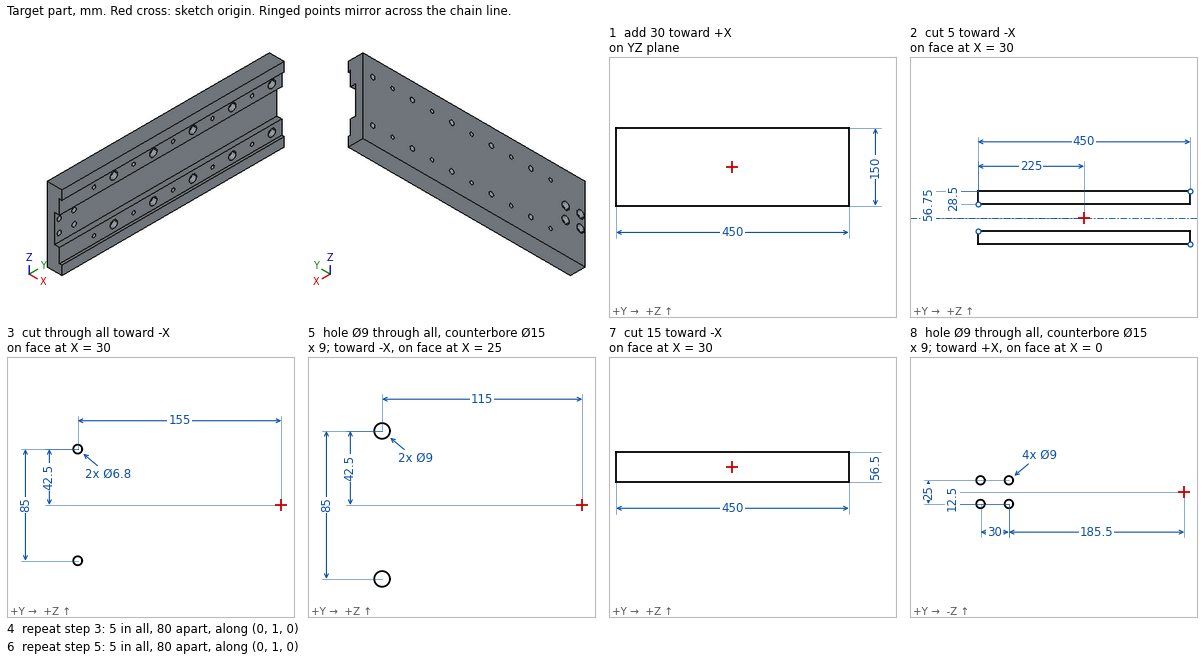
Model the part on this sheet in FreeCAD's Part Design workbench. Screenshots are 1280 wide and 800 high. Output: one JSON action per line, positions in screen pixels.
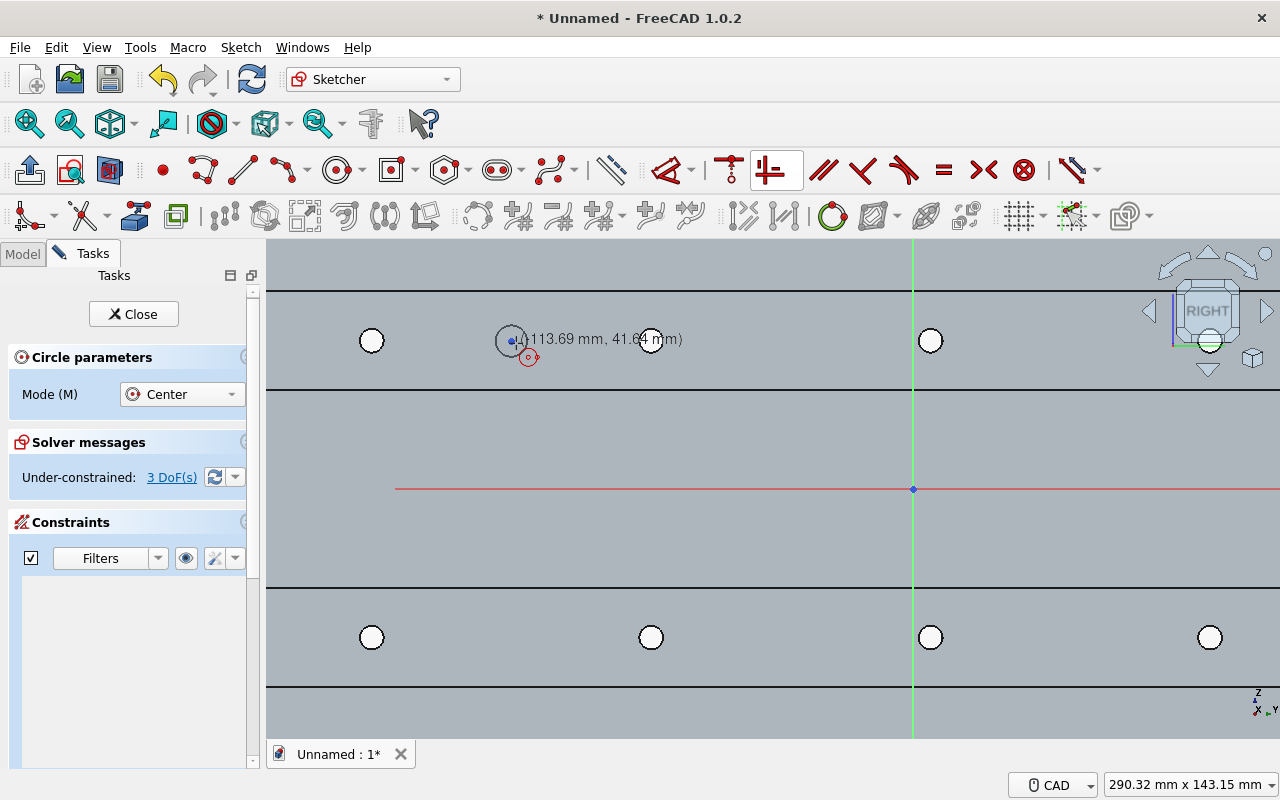
{"action": "scroll", "coordinate": [511, 638], "scroll_direction": "up", "scroll_amount": 2}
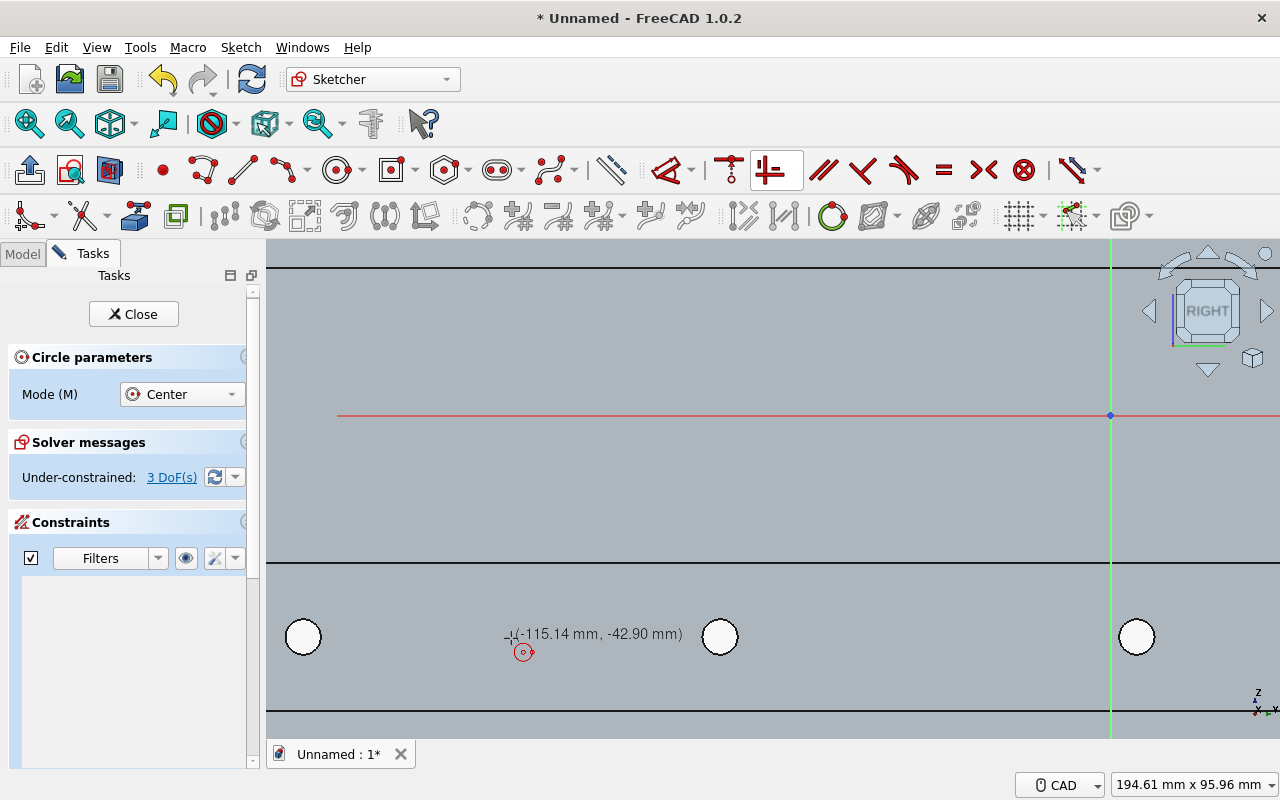
{"action": "left_click", "coordinate": [512, 637]}
{"action": "left_click", "coordinate": [528, 620]}
{"action": "key", "text": "Escape"}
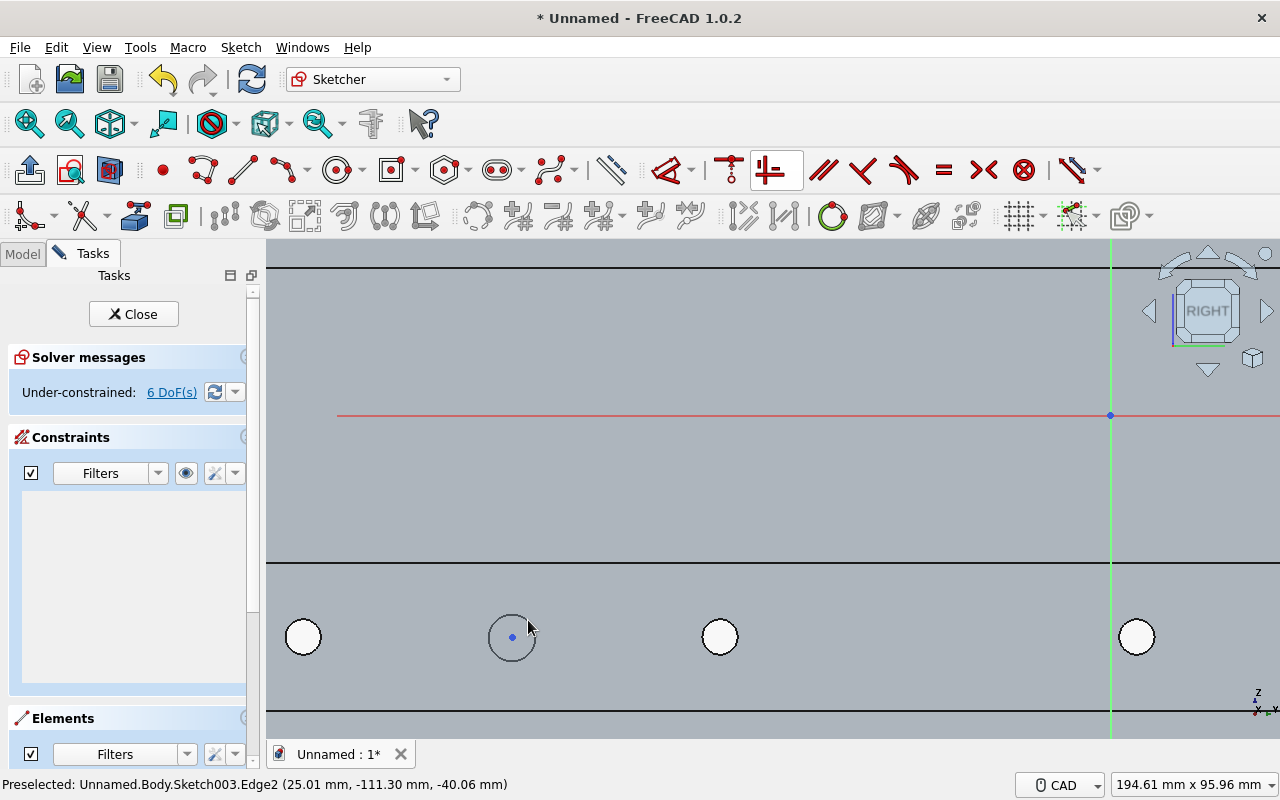
{"action": "scroll", "coordinate": [511, 638], "scroll_direction": "down", "scroll_amount": 2}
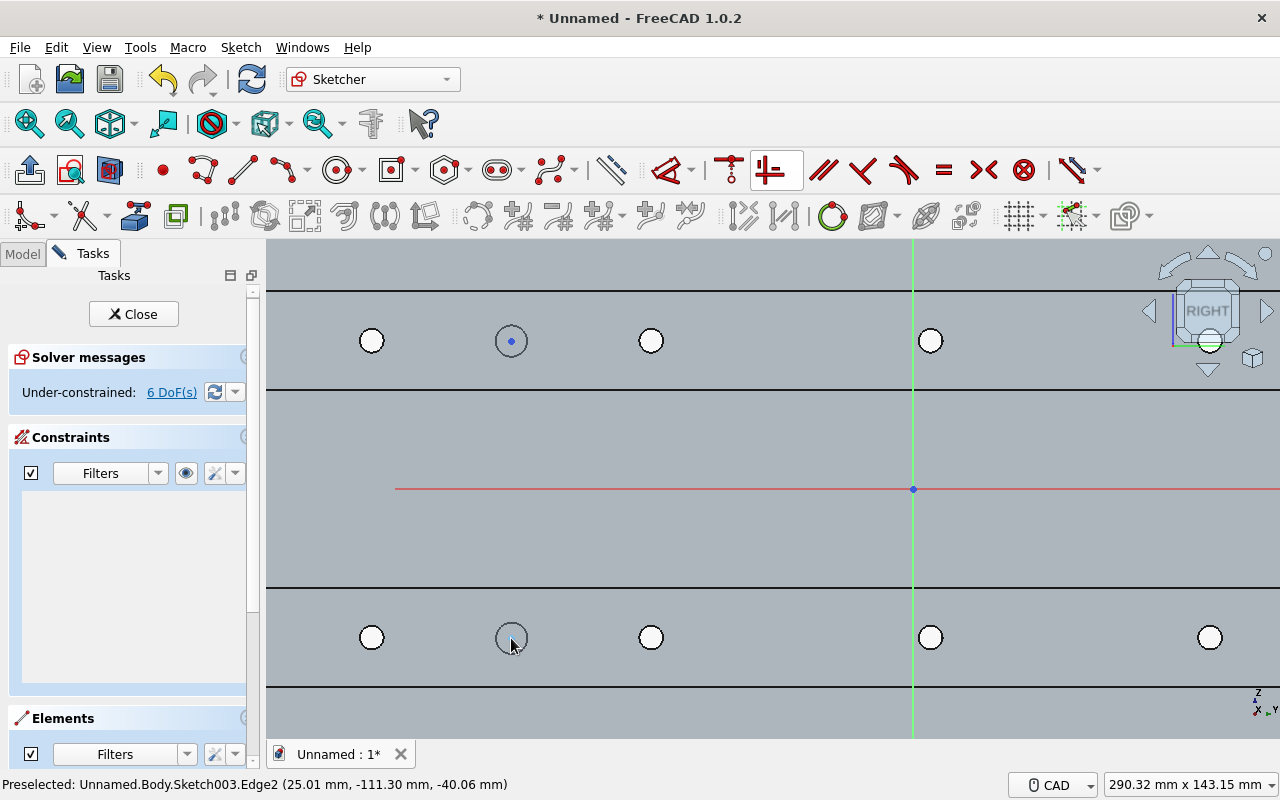
{"action": "left_click", "coordinate": [522, 330]}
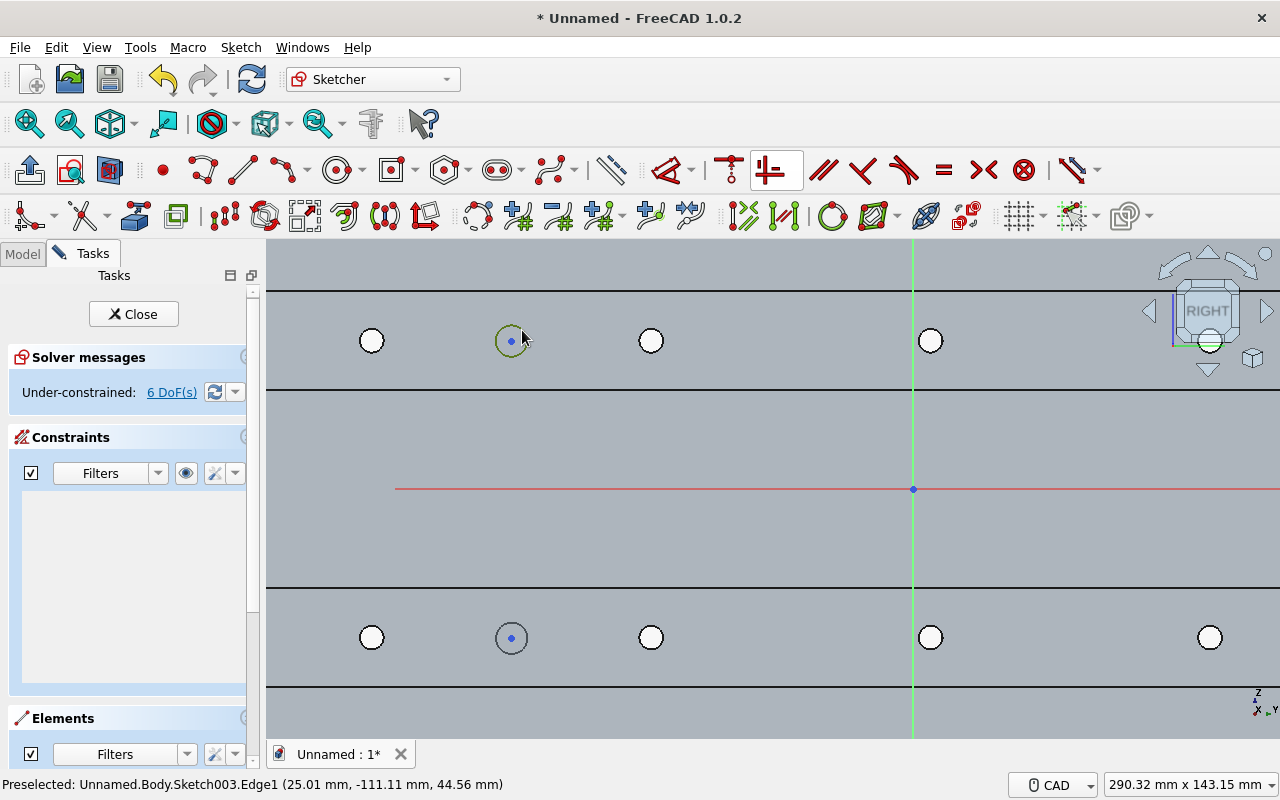
{"action": "left_click", "coordinate": [523, 627]}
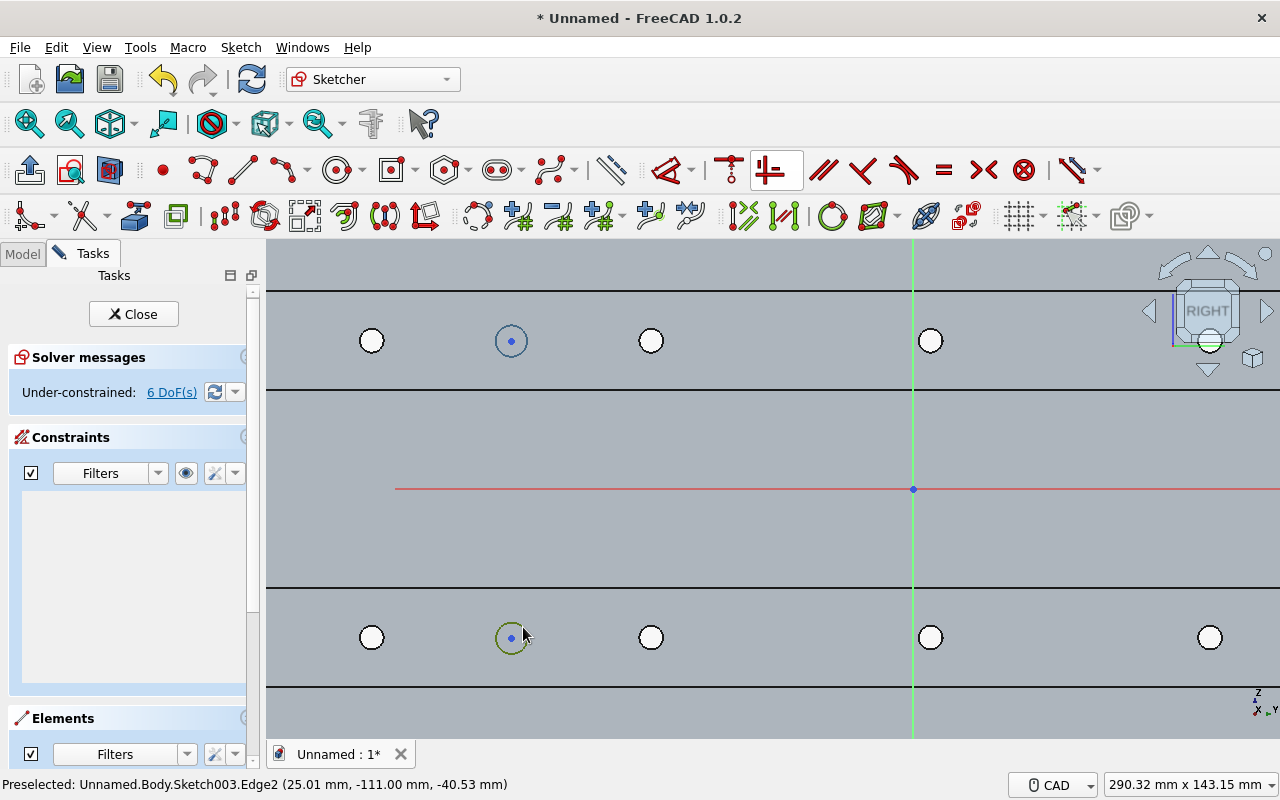
{"action": "left_click", "coordinate": [944, 170]}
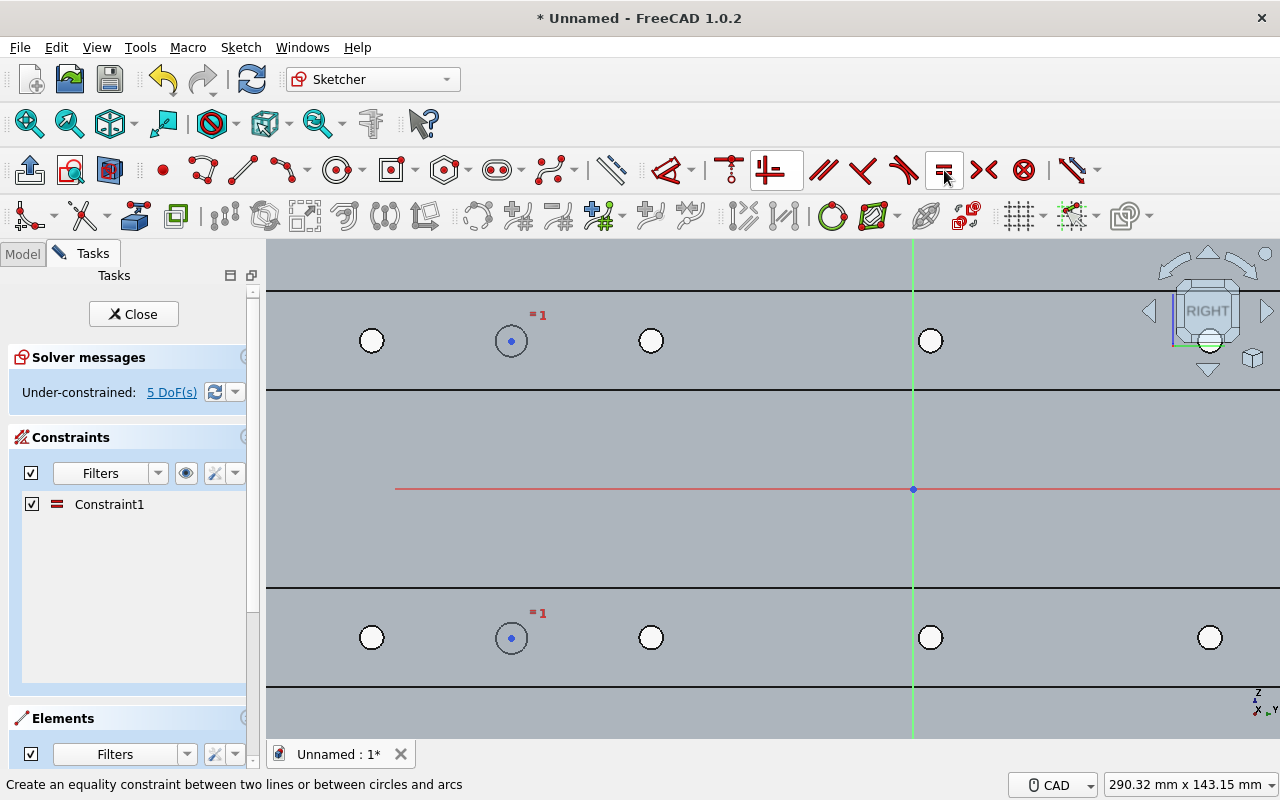
{"action": "left_click", "coordinate": [511, 341]}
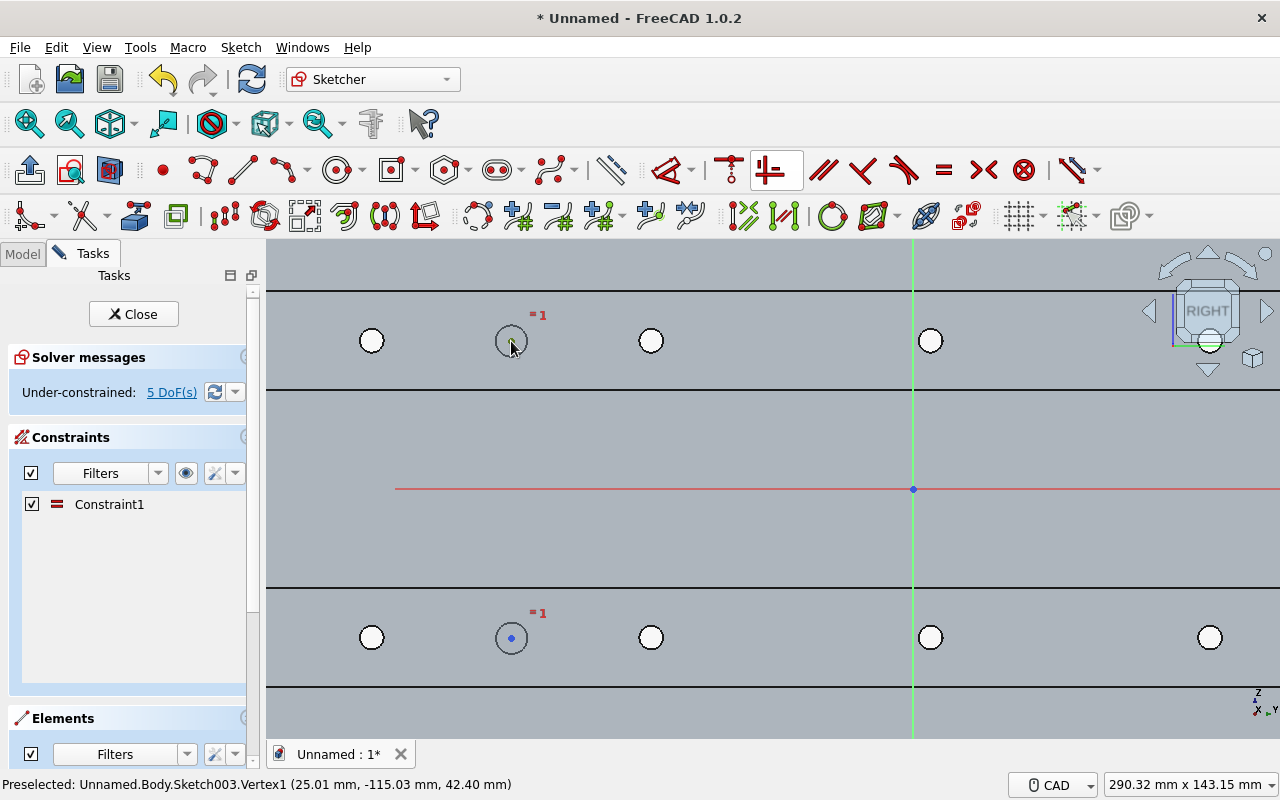
{"action": "left_click", "coordinate": [512, 638]}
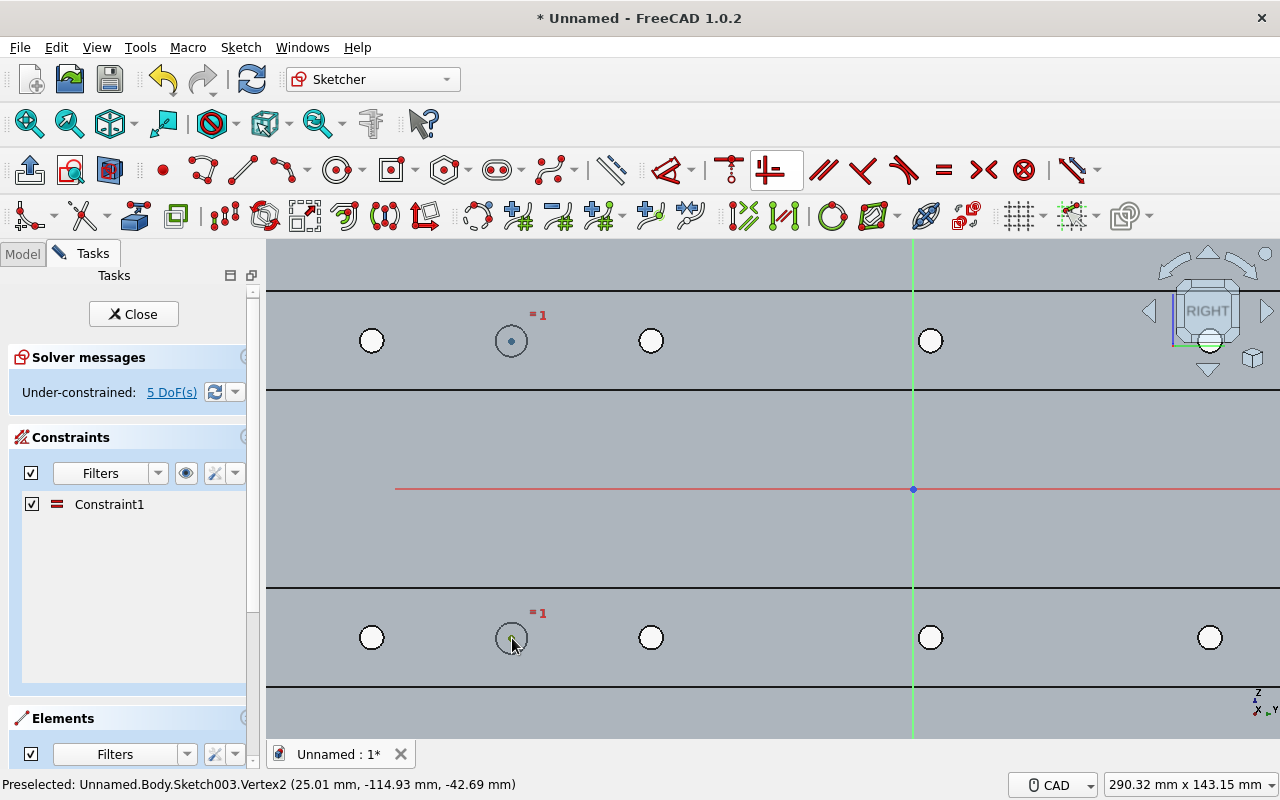
{"action": "left_click", "coordinate": [798, 170]}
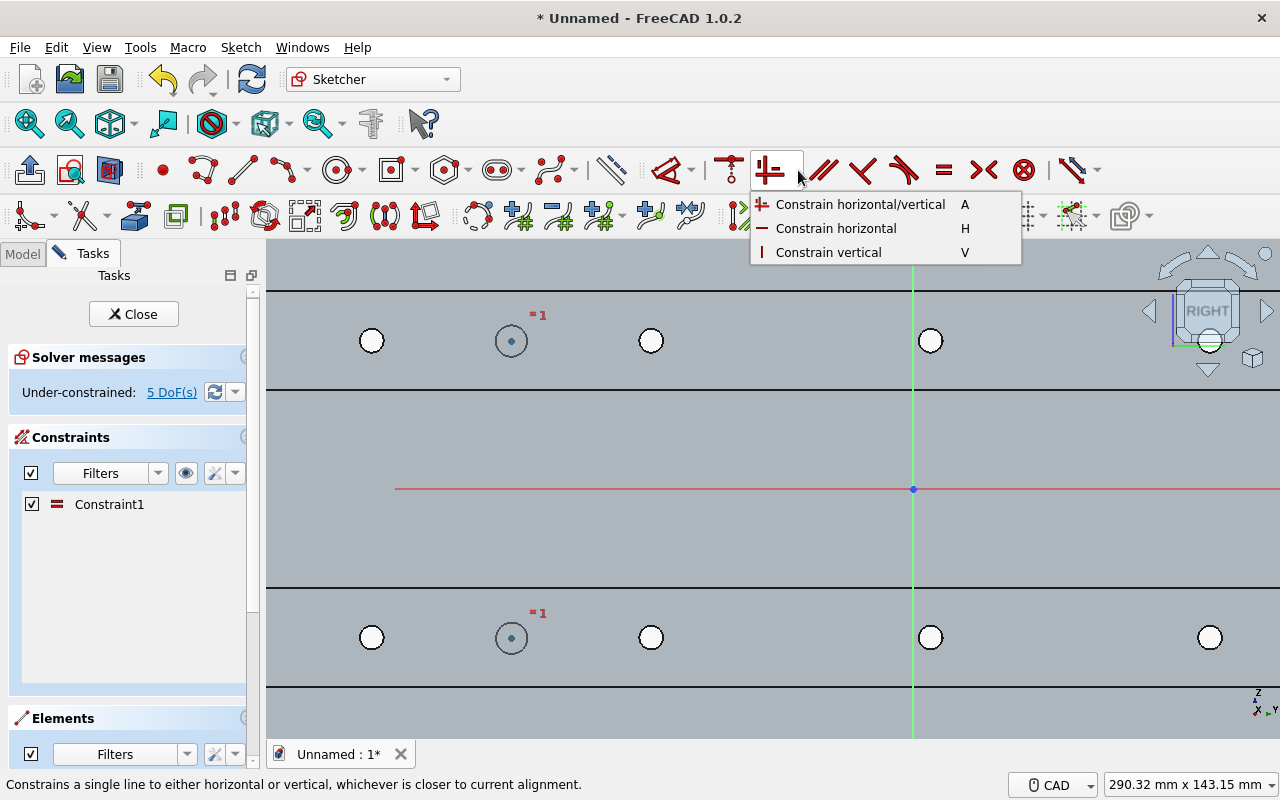
{"action": "left_click", "coordinate": [886, 252]}